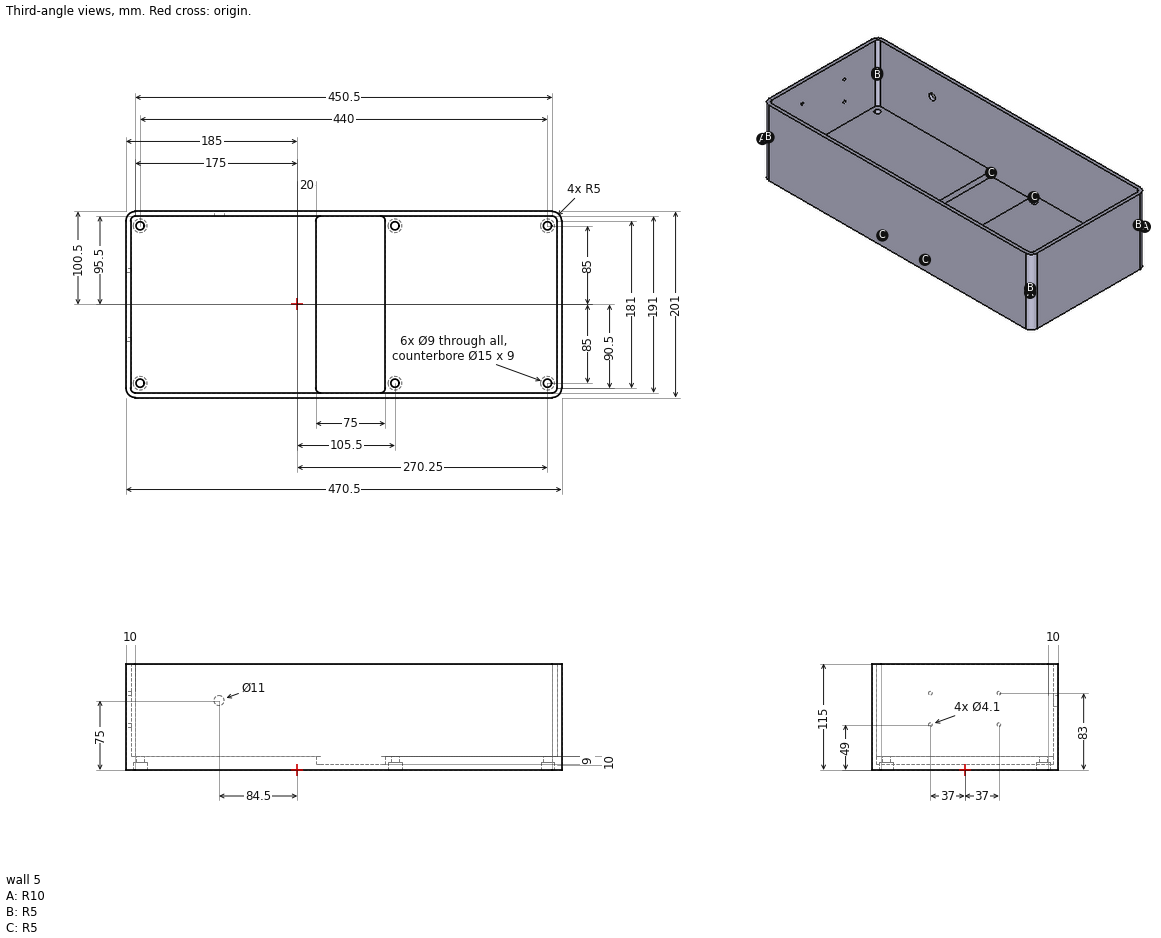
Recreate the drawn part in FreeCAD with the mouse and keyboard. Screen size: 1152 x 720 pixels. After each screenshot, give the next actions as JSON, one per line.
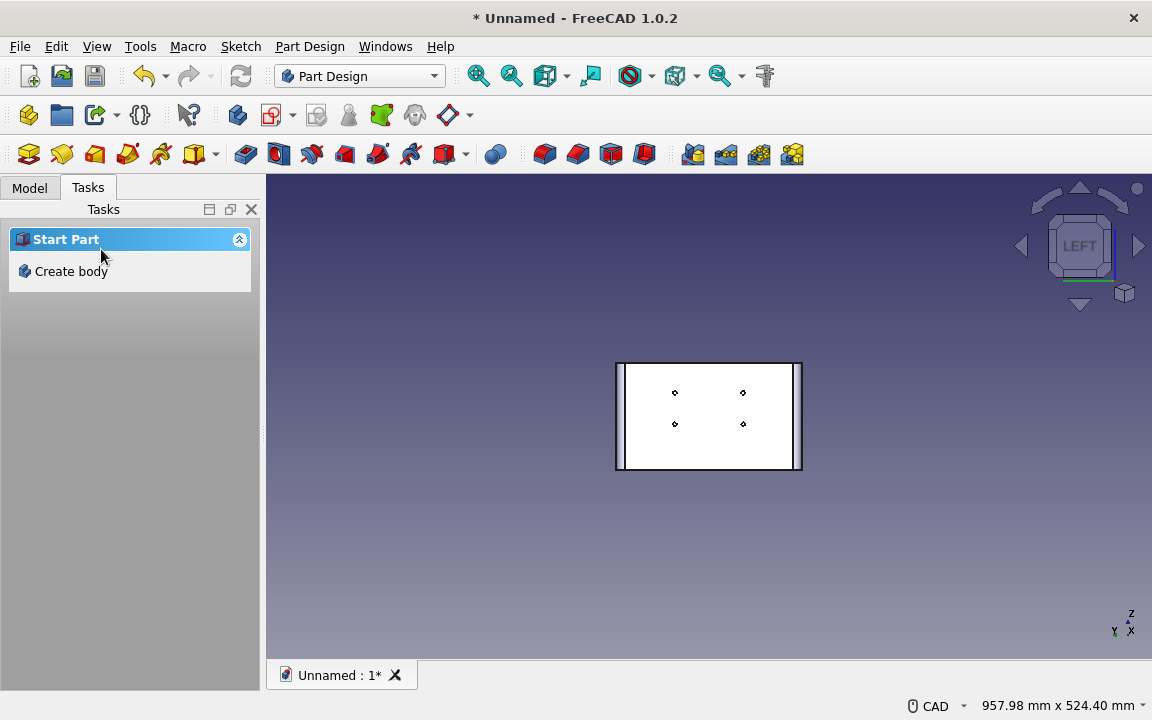
{"action": "key", "text": "0"}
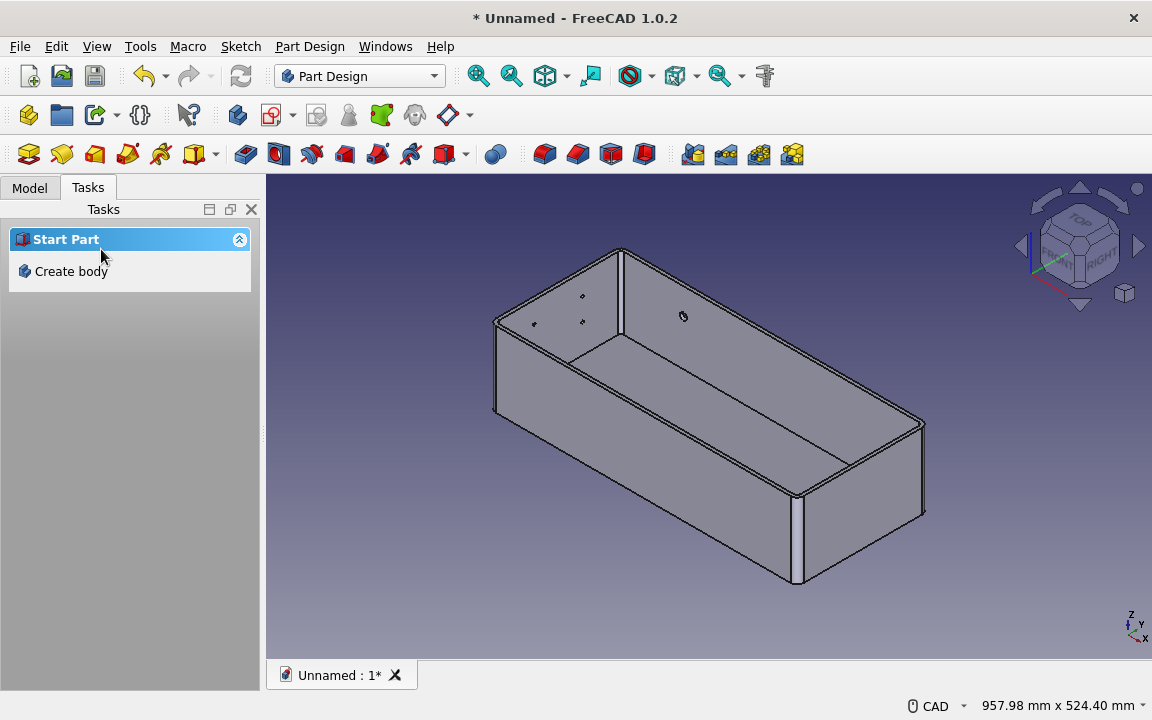
{"action": "key", "text": "2"}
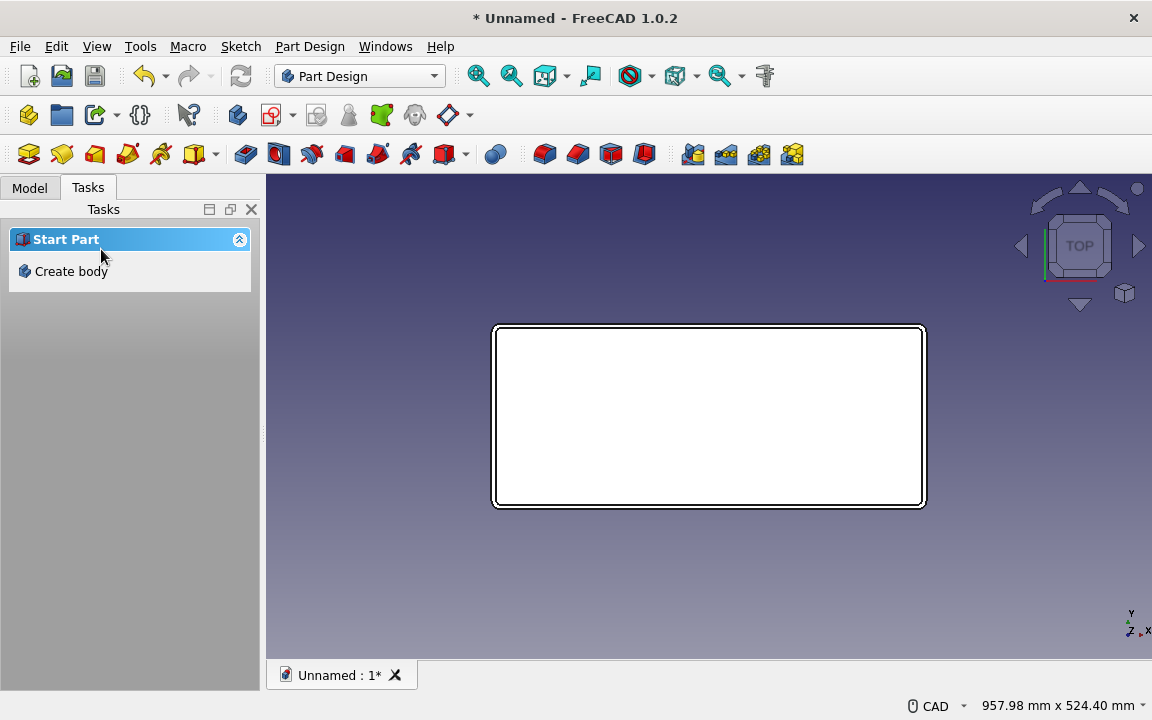
{"action": "left_click", "coordinate": [831, 415]}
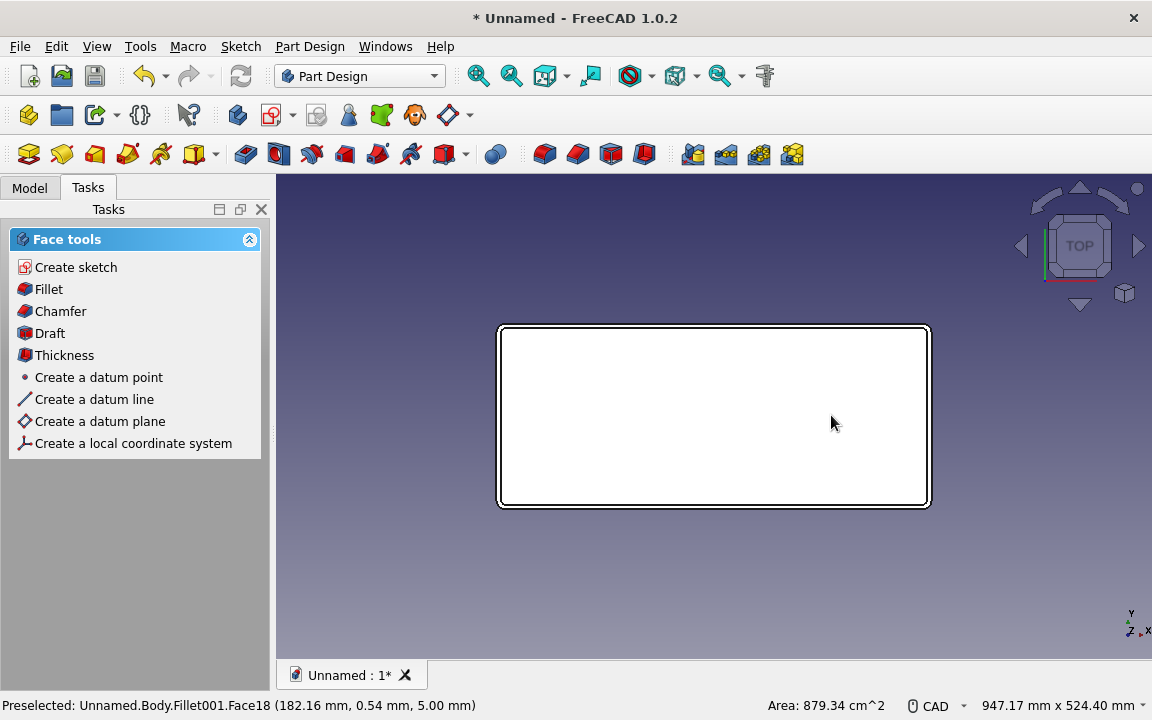
{"action": "left_click", "coordinate": [270, 116]}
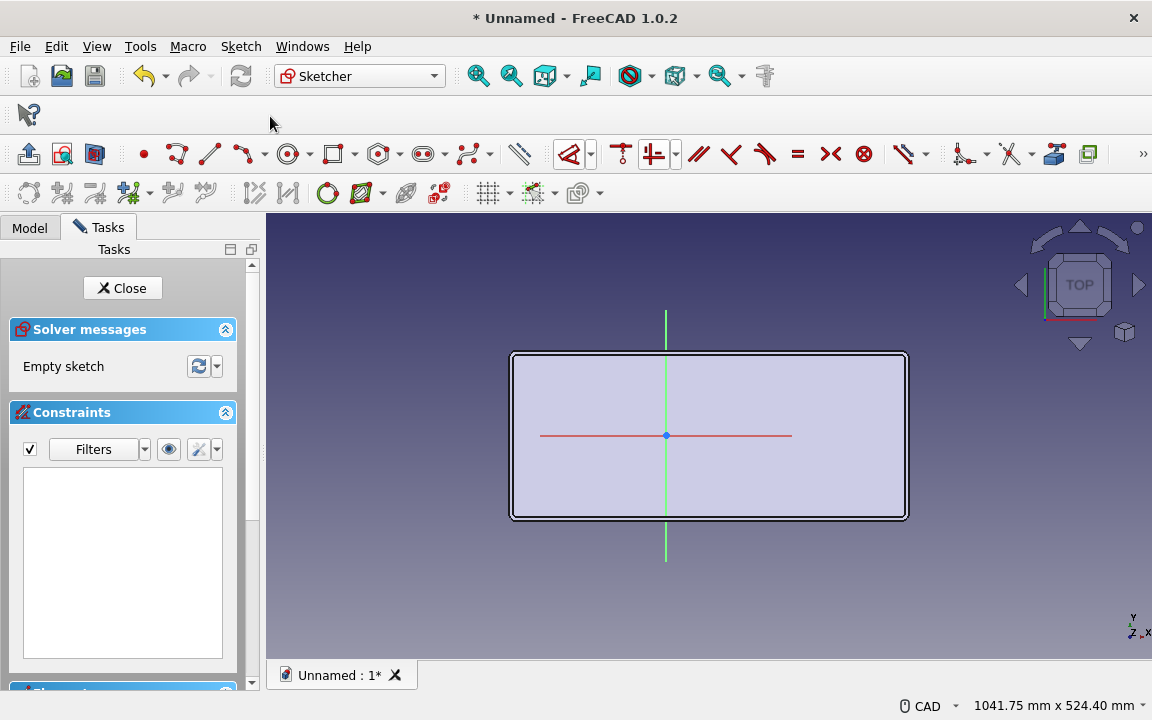
{"action": "key", "text": "g l"}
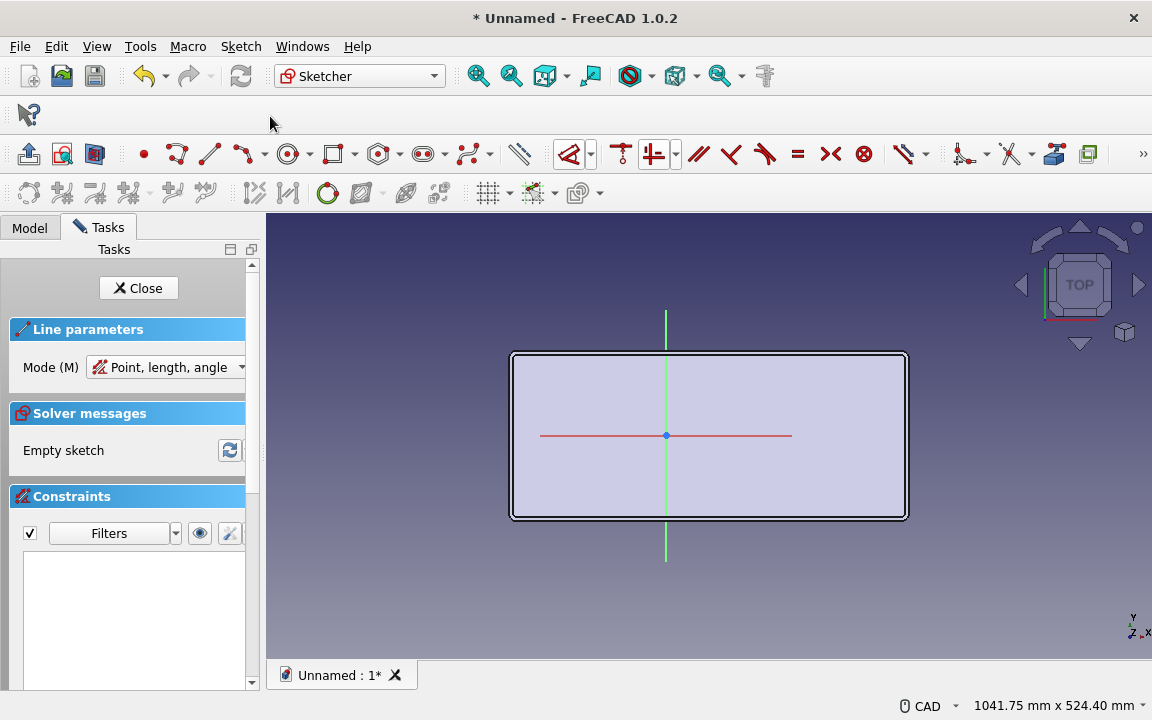
{"action": "left_click", "coordinate": [905, 513]}
{"action": "left_click", "coordinate": [905, 359]}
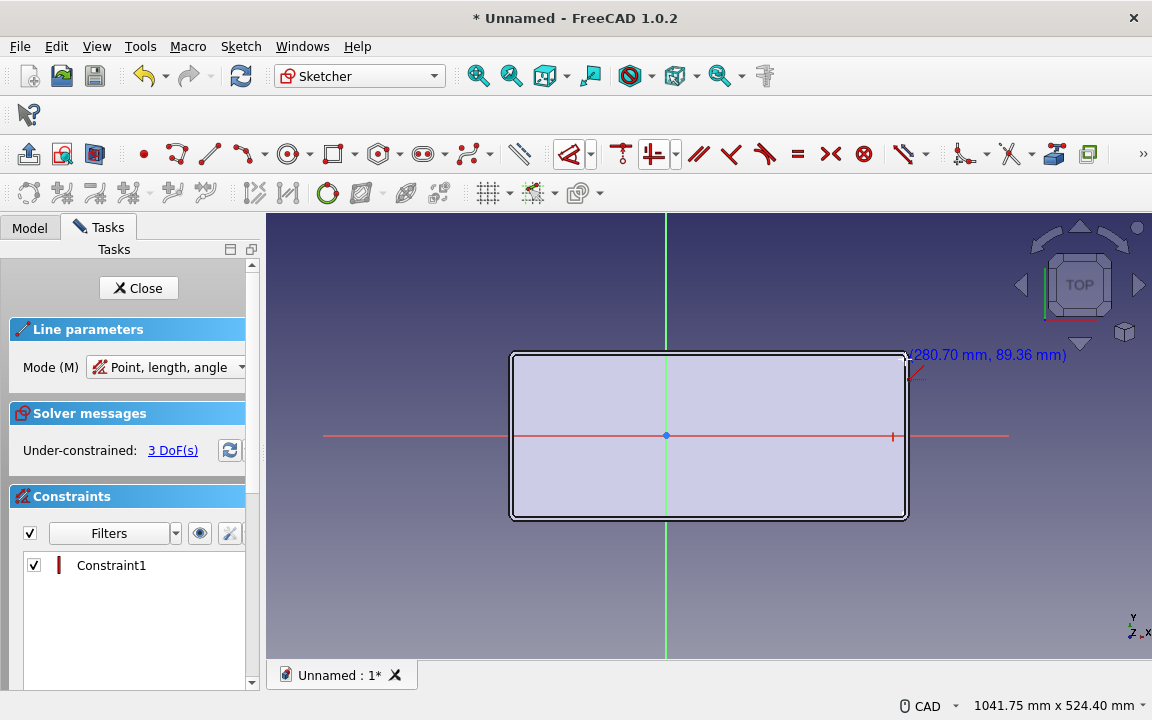
{"action": "scroll", "coordinate": [901, 355], "scroll_direction": "up", "scroll_amount": 5}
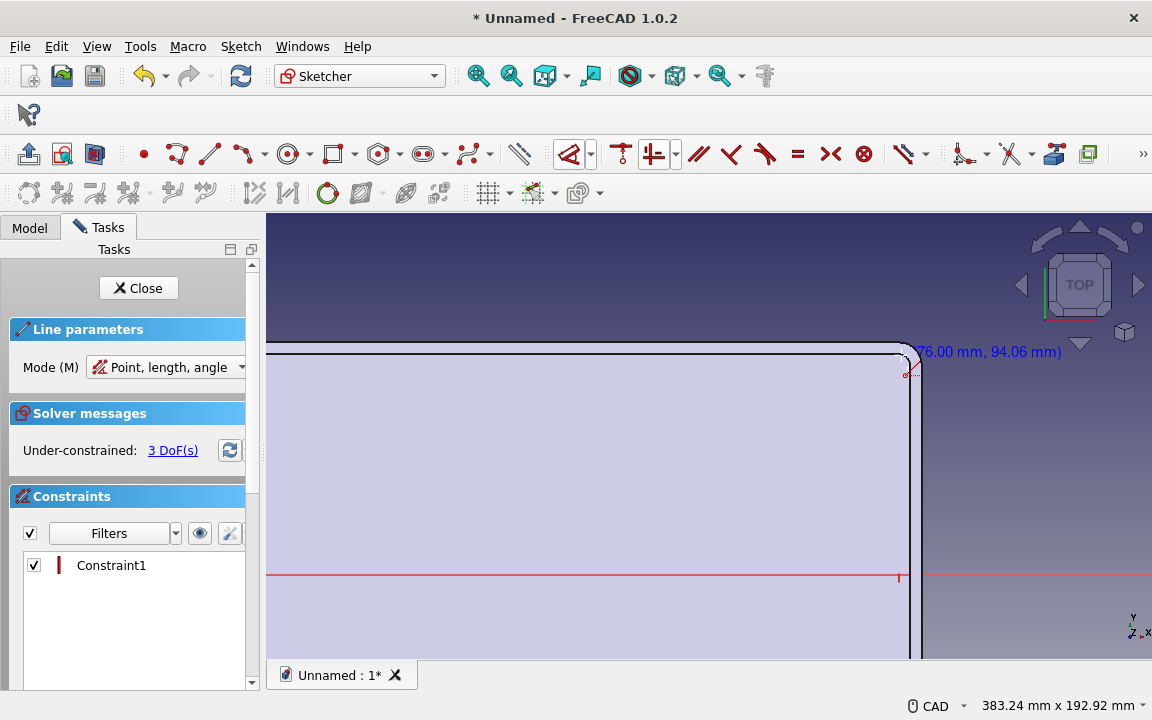
{"action": "left_click", "coordinate": [899, 354]}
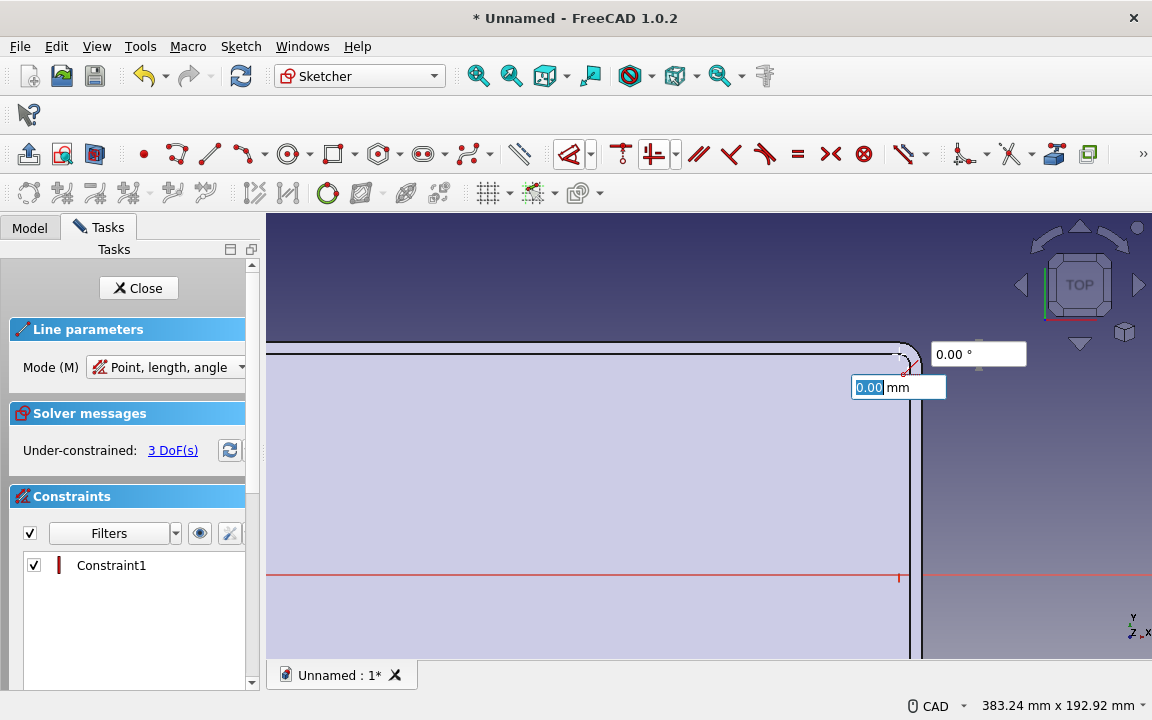
{"action": "scroll", "coordinate": [855, 323], "scroll_direction": "down", "scroll_amount": 4}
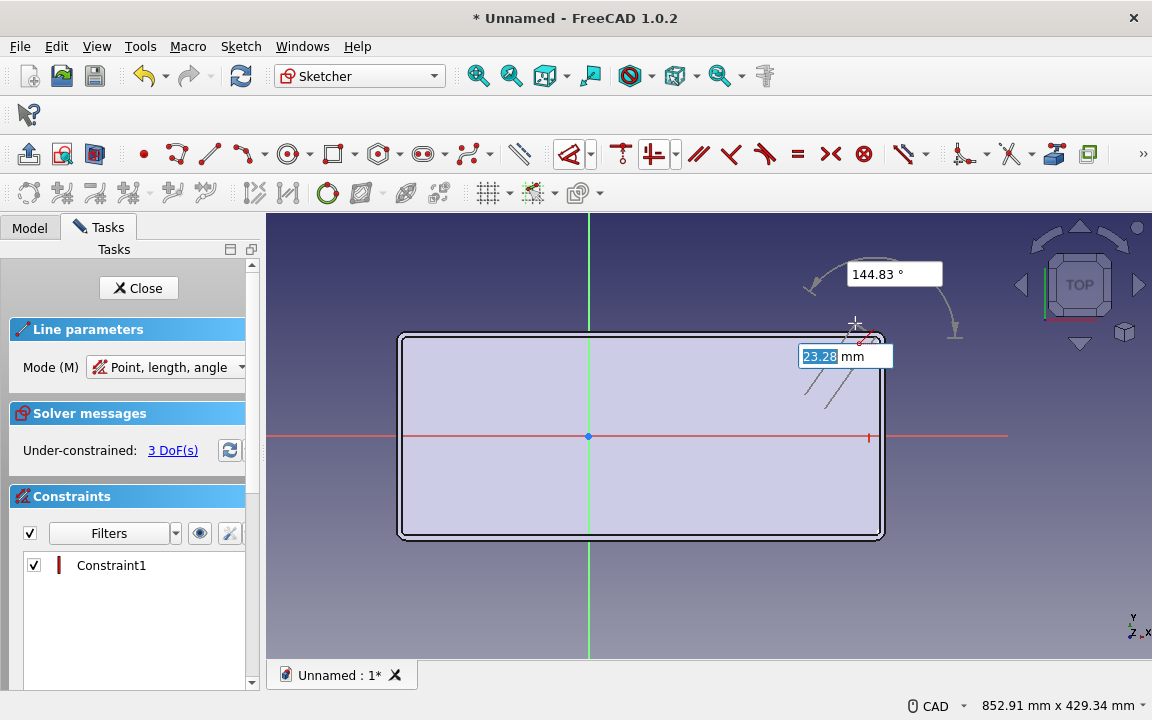
{"action": "left_click", "coordinate": [407, 337]}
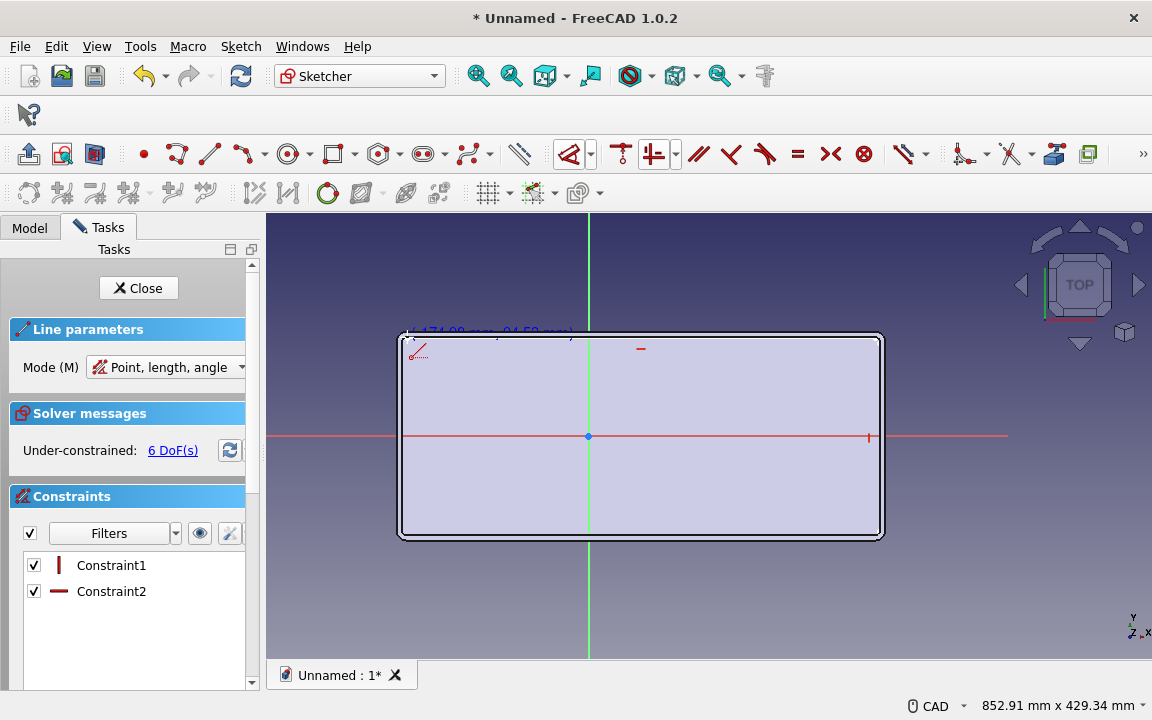
{"action": "scroll", "coordinate": [402, 342], "scroll_direction": "up", "scroll_amount": 4}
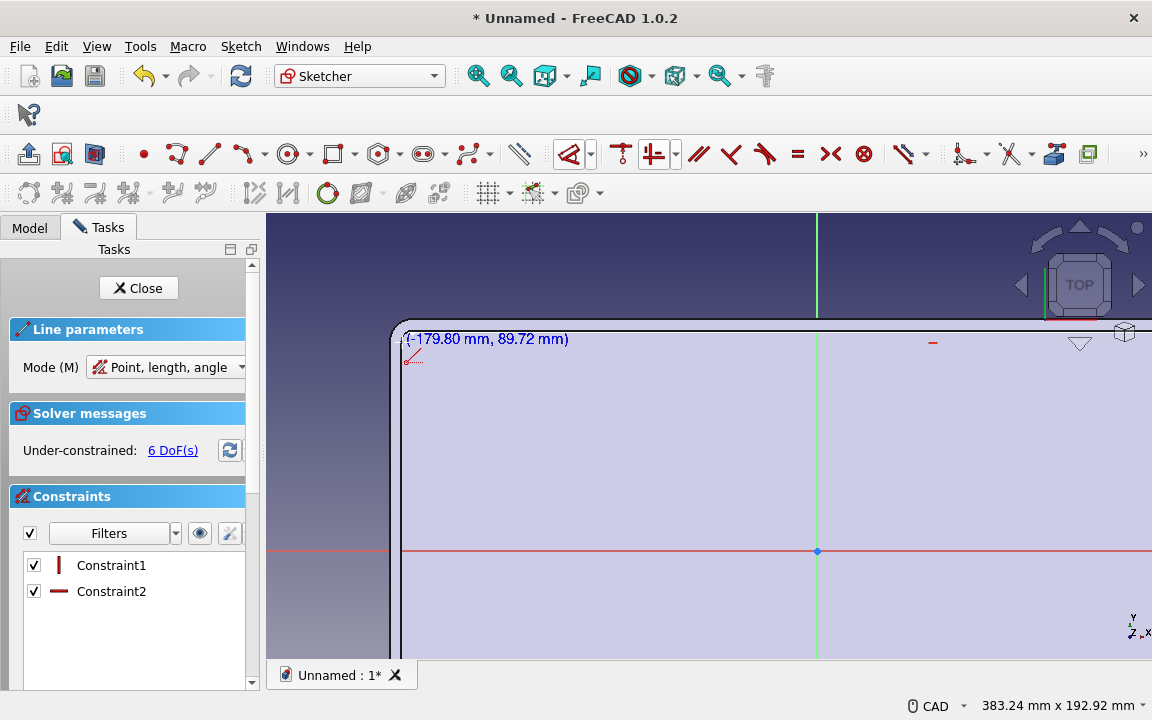
{"action": "left_click", "coordinate": [401, 342]}